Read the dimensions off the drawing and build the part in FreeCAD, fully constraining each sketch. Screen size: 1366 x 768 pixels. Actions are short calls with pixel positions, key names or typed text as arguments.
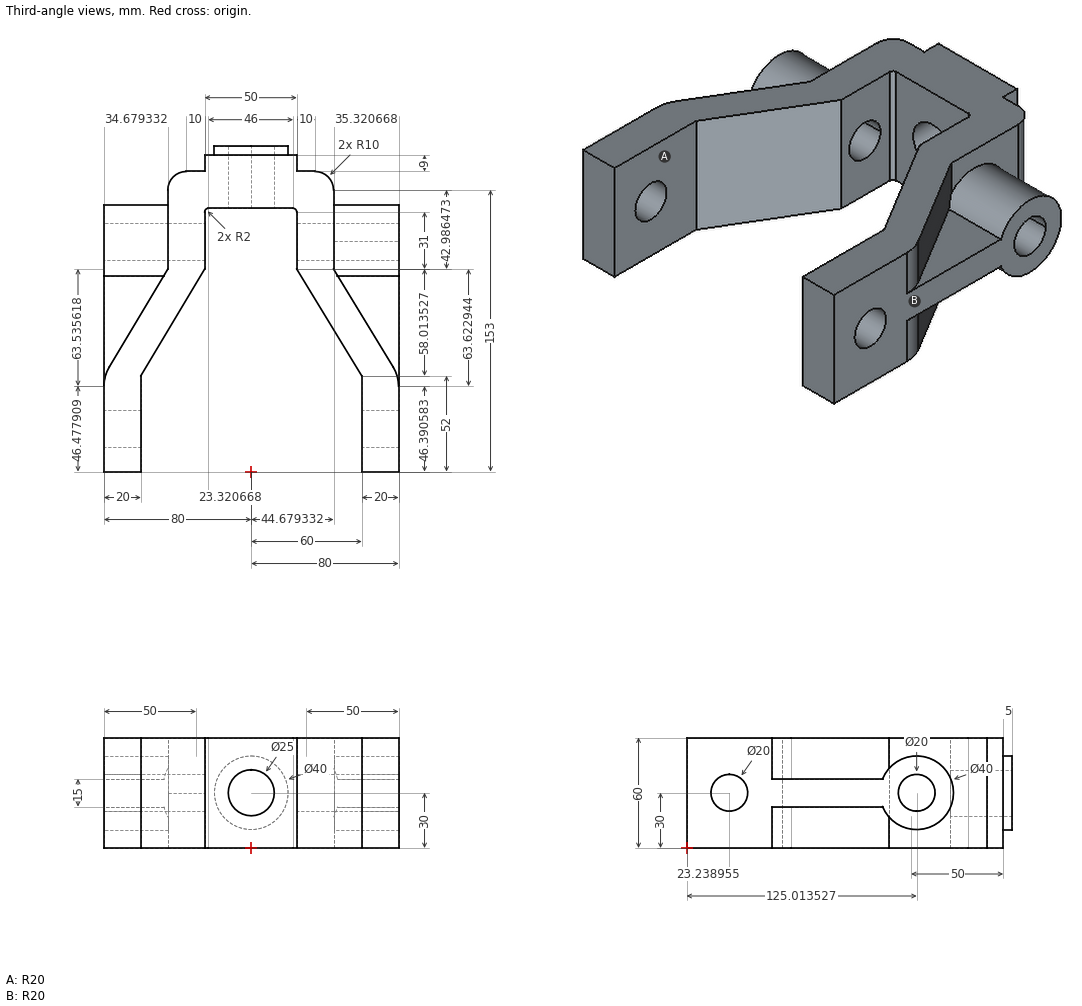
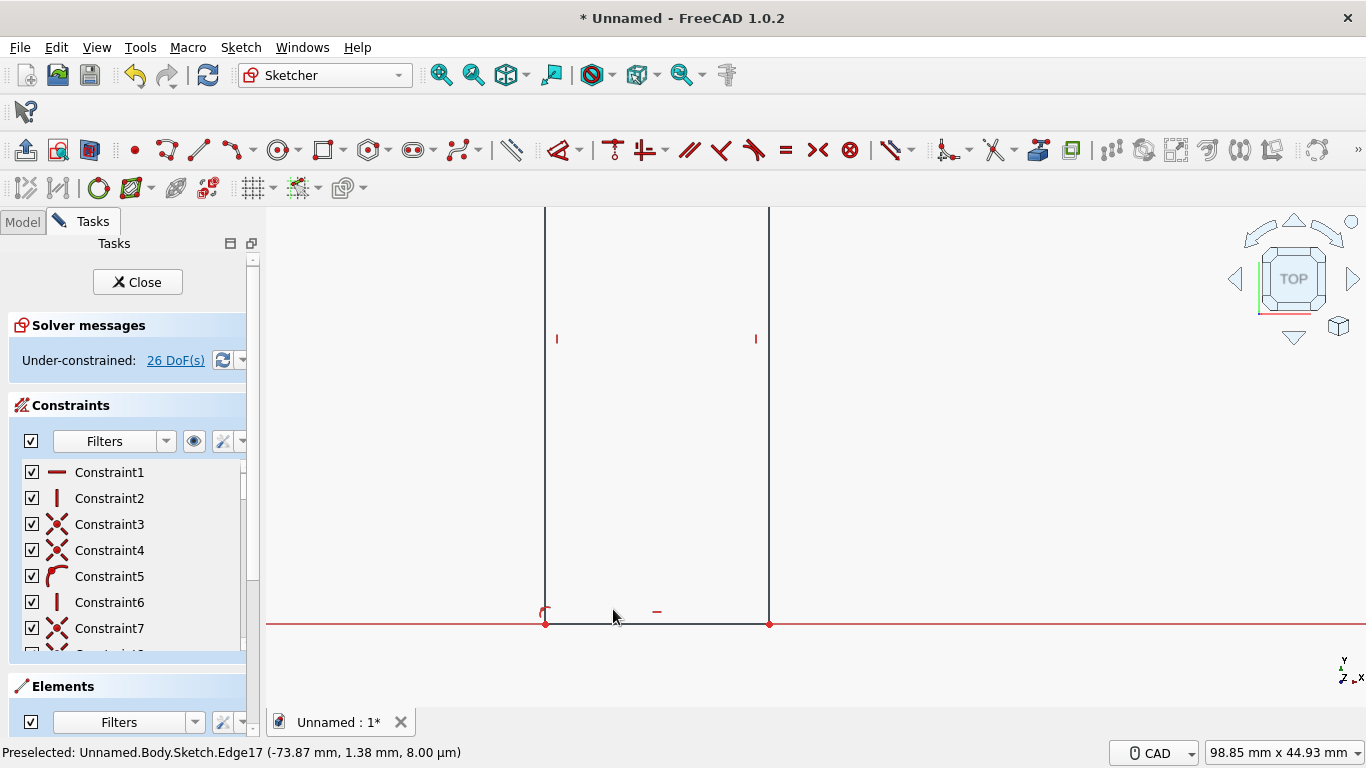
scroll(611, 613, down, 9)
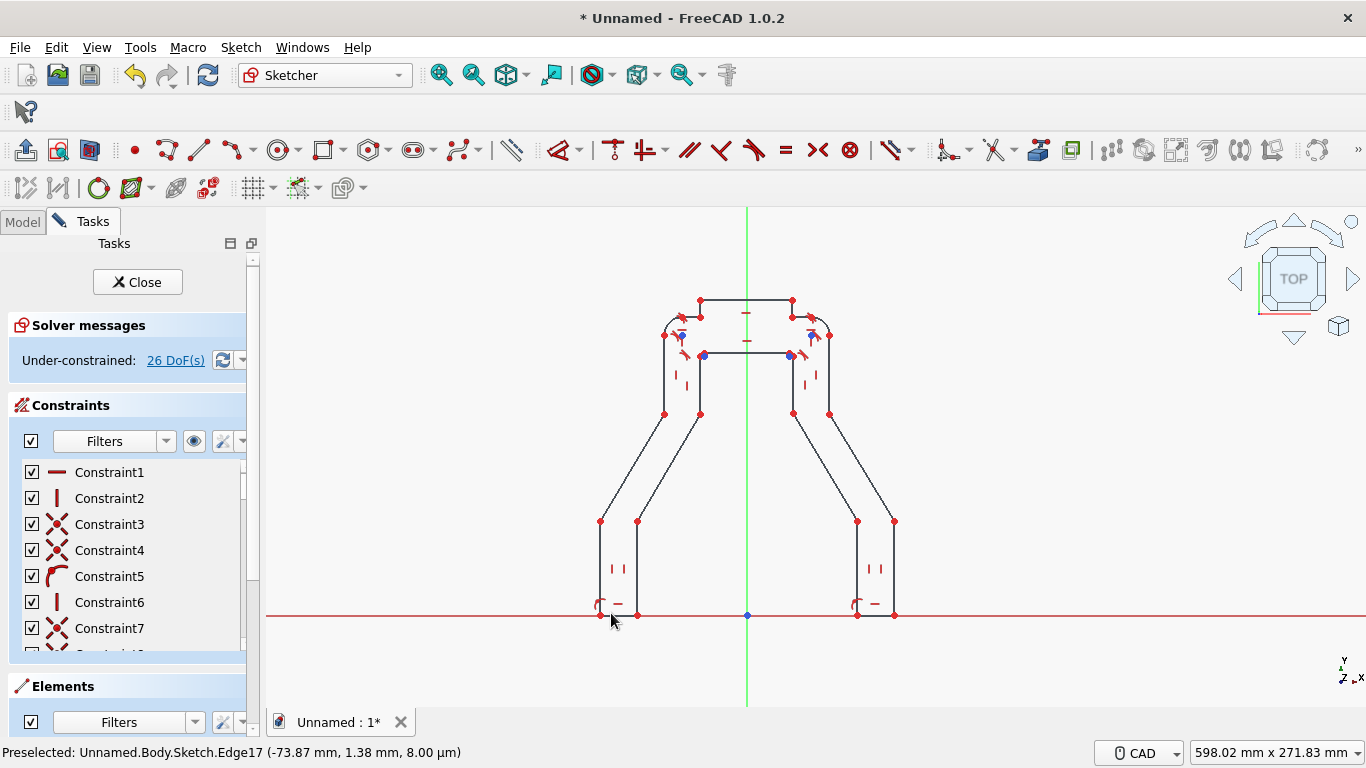
scroll(827, 327, up, 3)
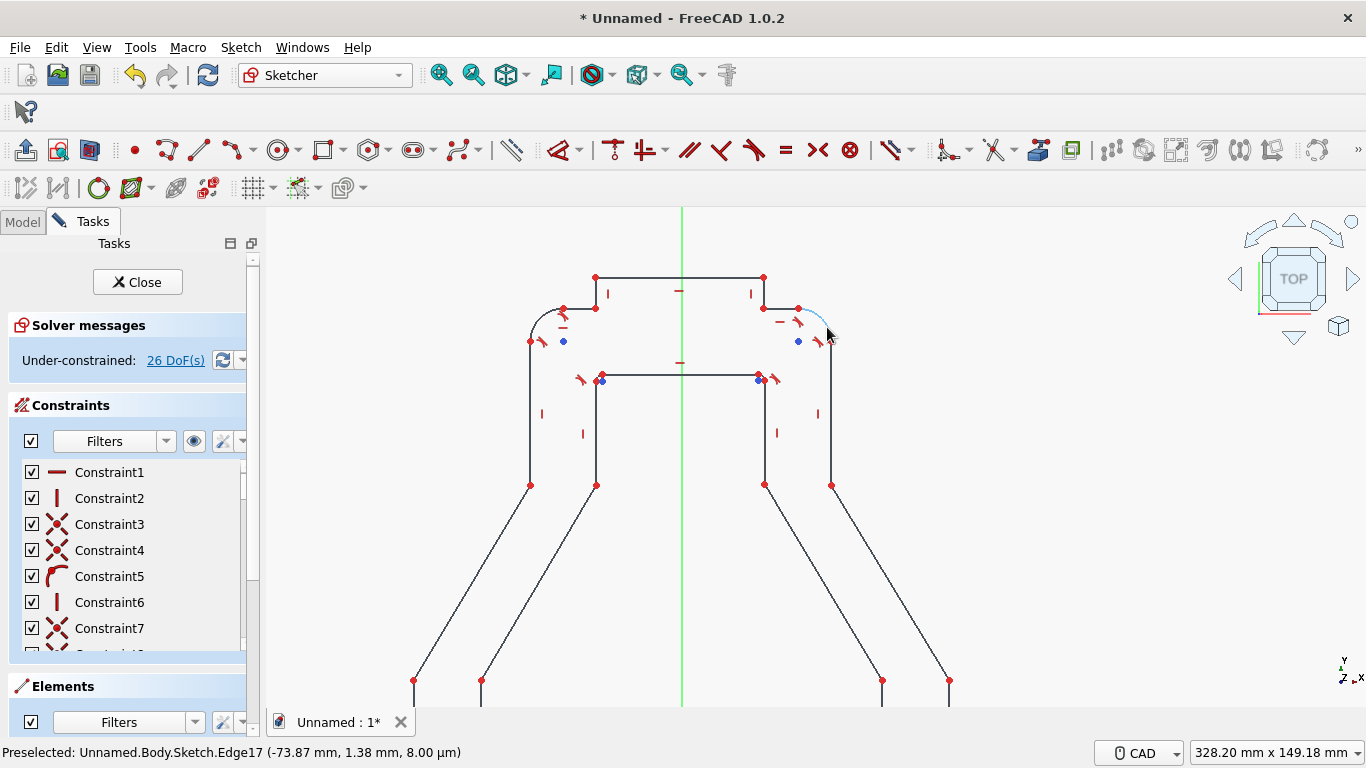
click(827, 327)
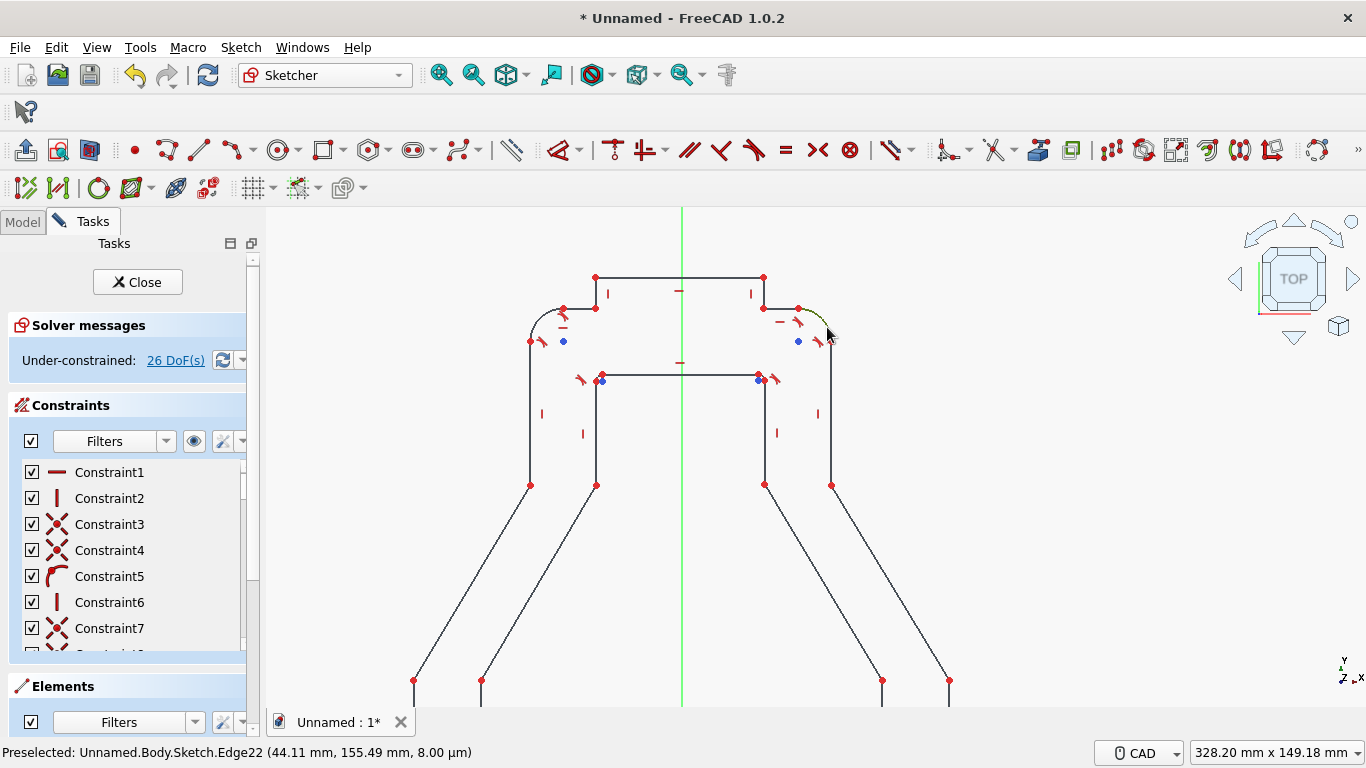
click(548, 312)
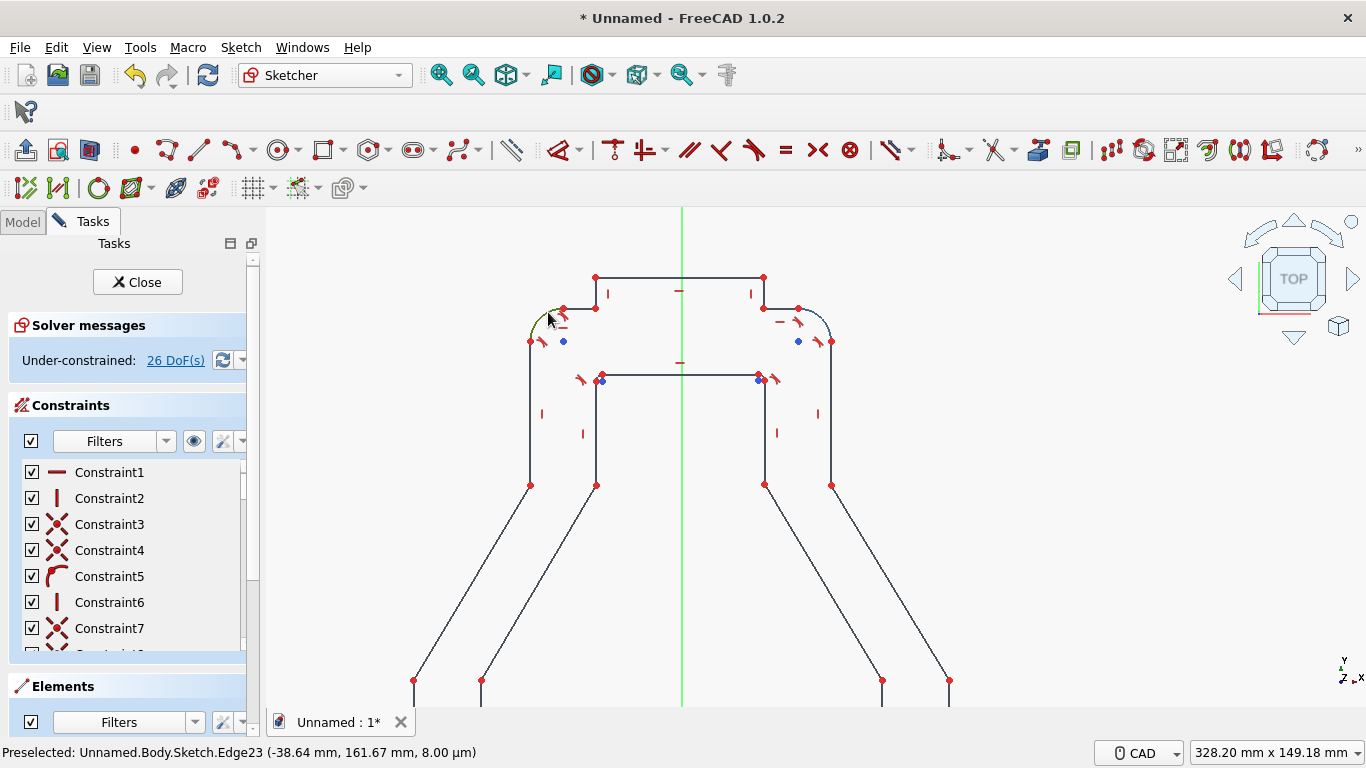
click(786, 150)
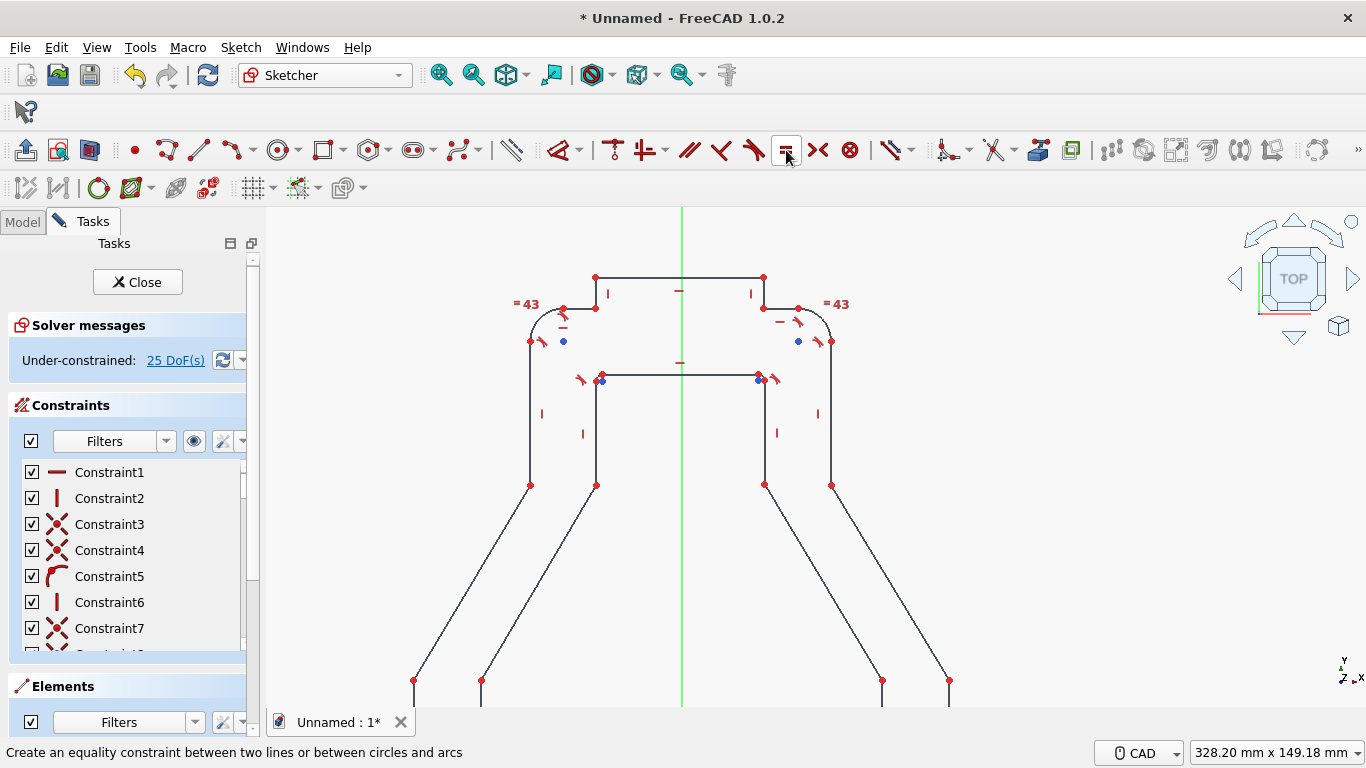
scroll(763, 376, up, 6)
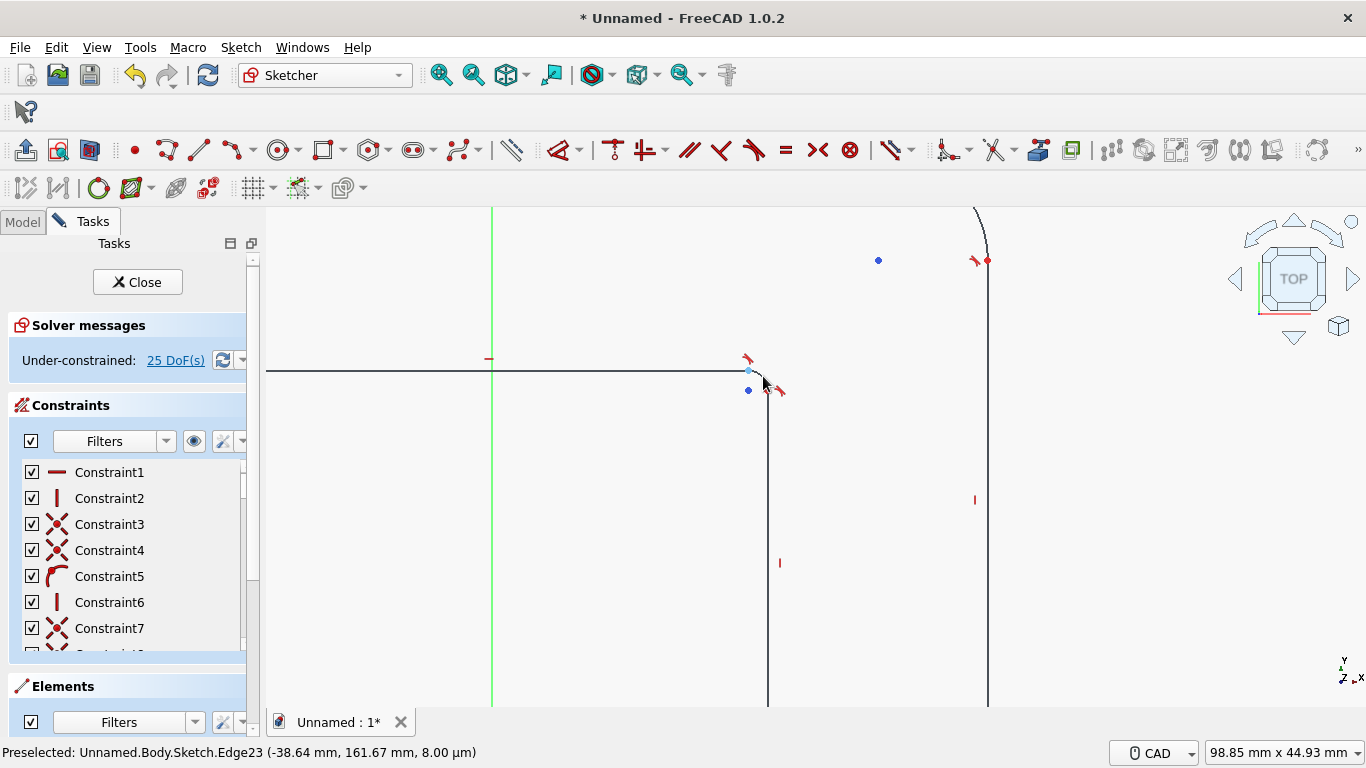
click(762, 376)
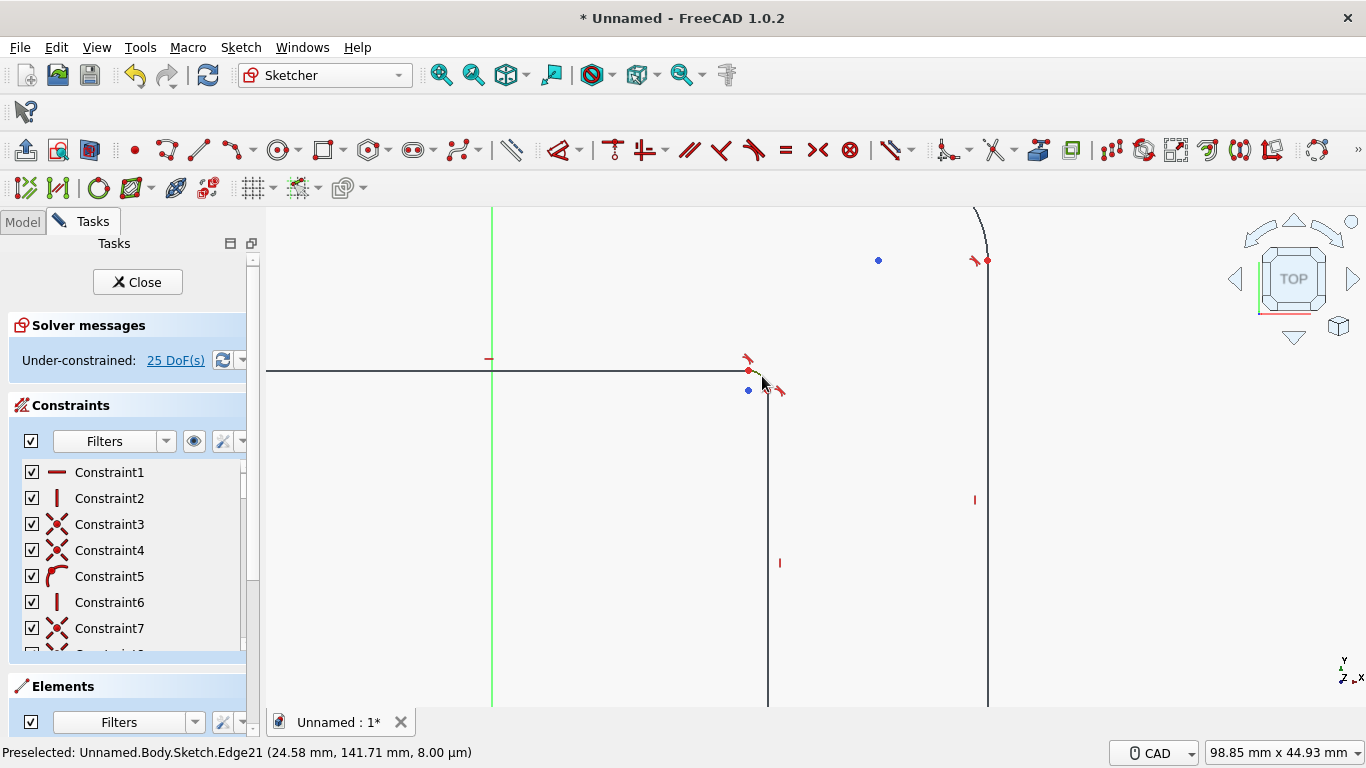
scroll(798, 349, down, 9)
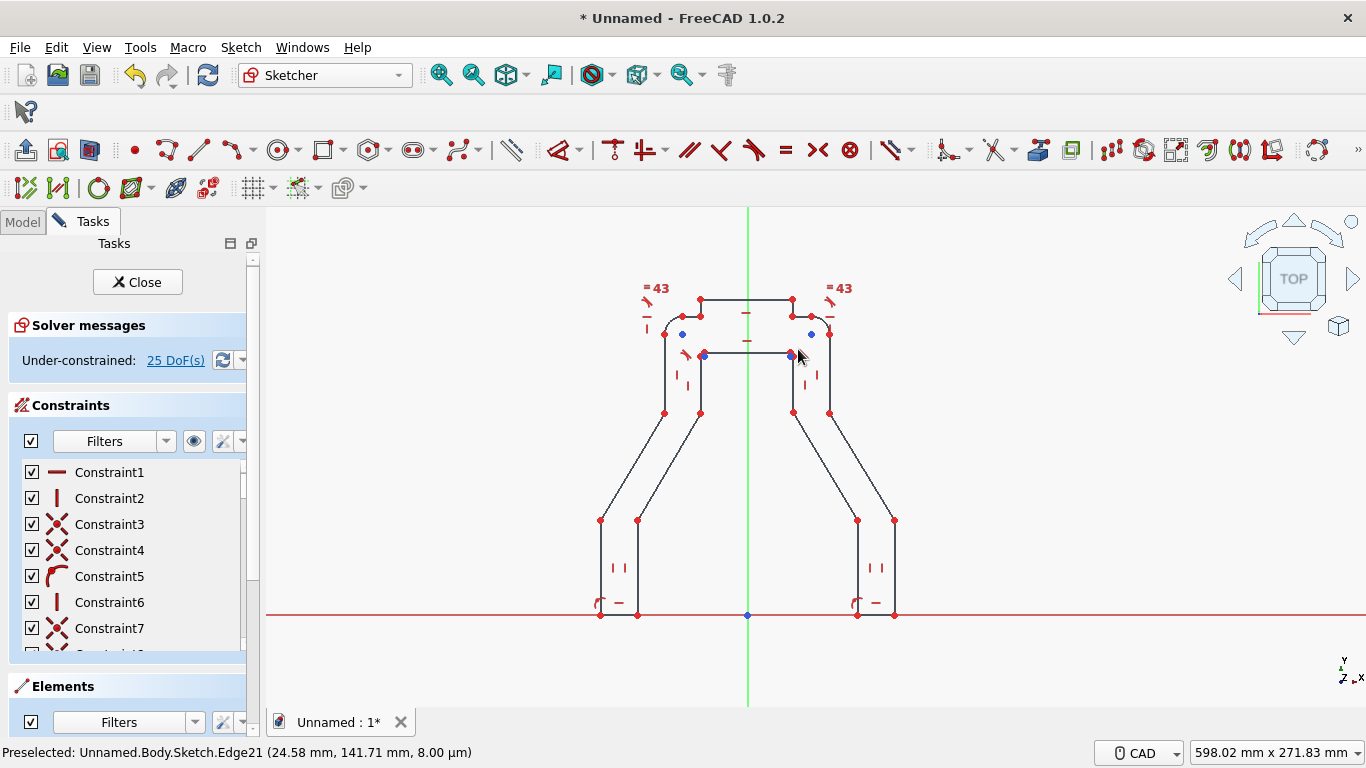
scroll(703, 353, up, 11)